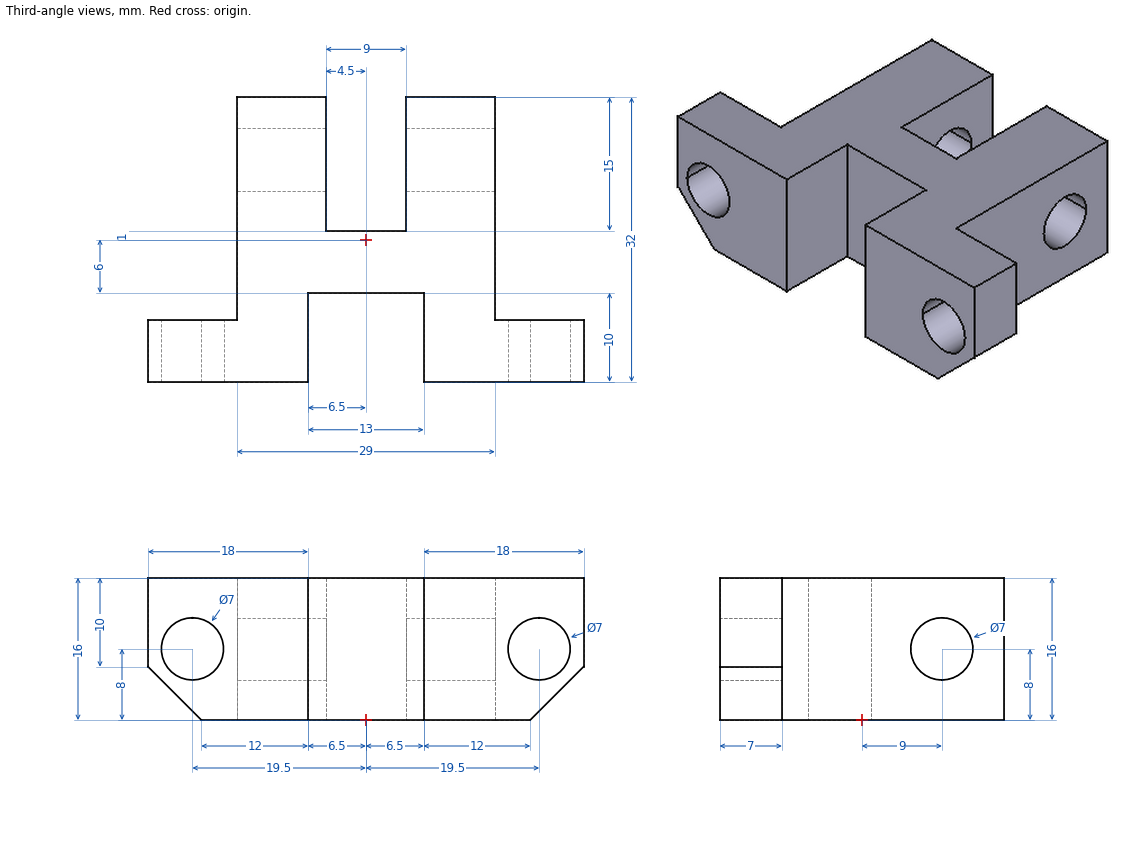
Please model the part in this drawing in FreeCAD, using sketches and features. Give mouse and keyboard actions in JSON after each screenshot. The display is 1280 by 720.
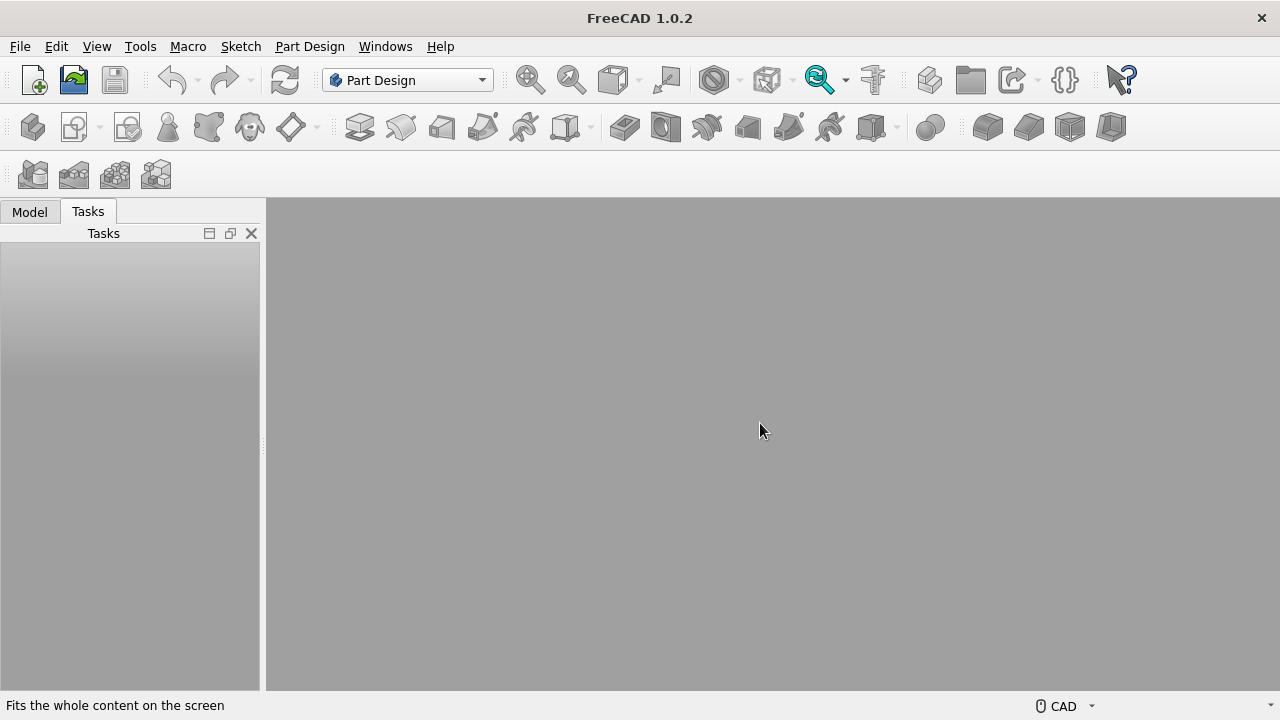
{"action": "left_click", "coordinate": [33, 80]}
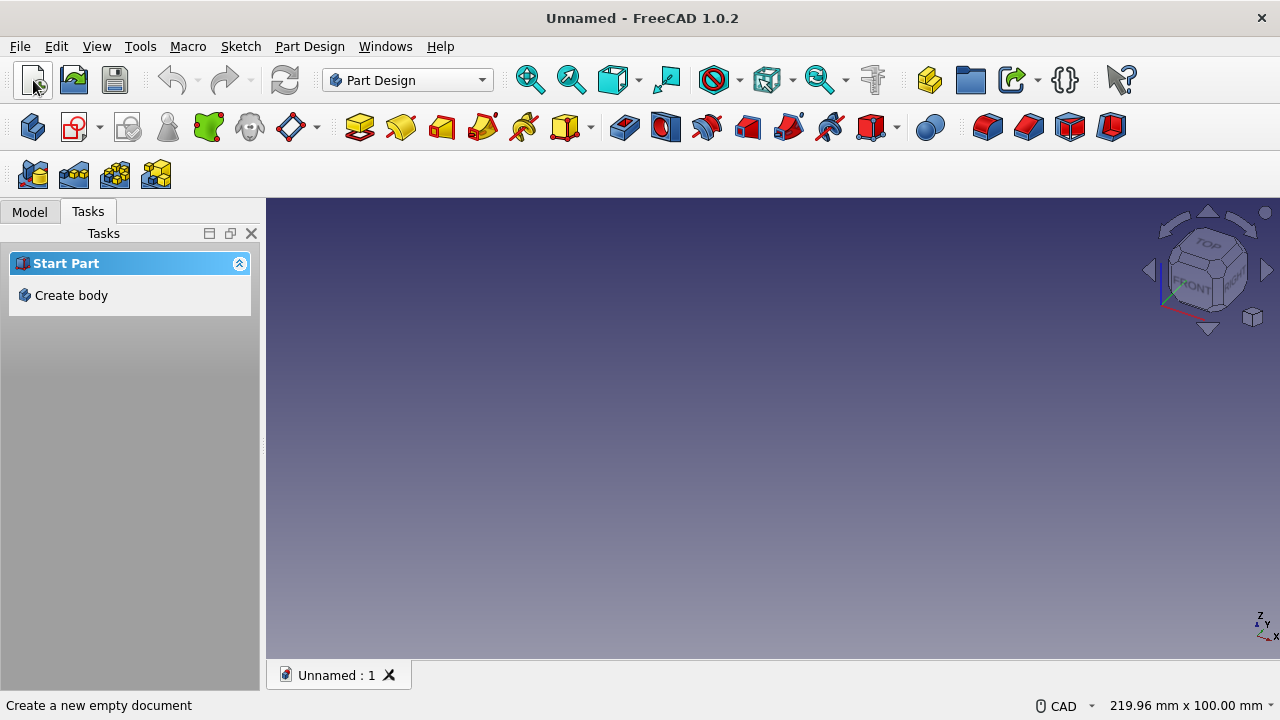
{"action": "left_click", "coordinate": [74, 128]}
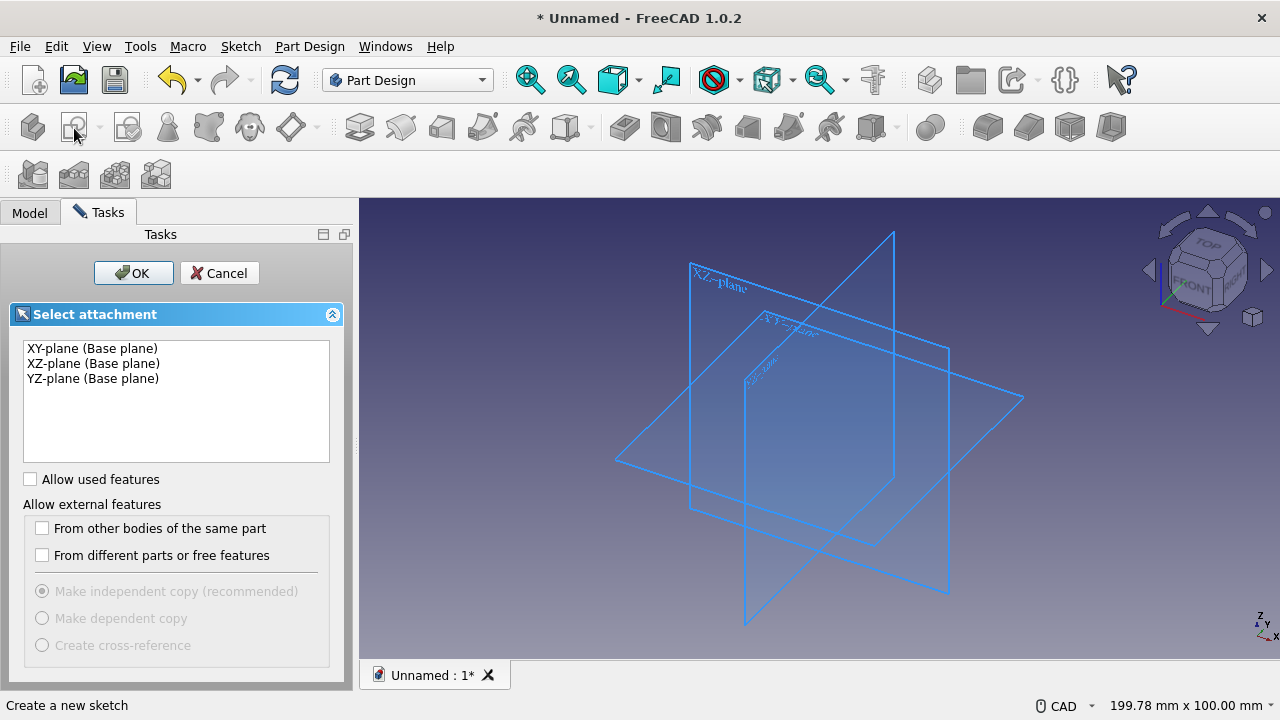
{"action": "left_click", "coordinate": [84, 348]}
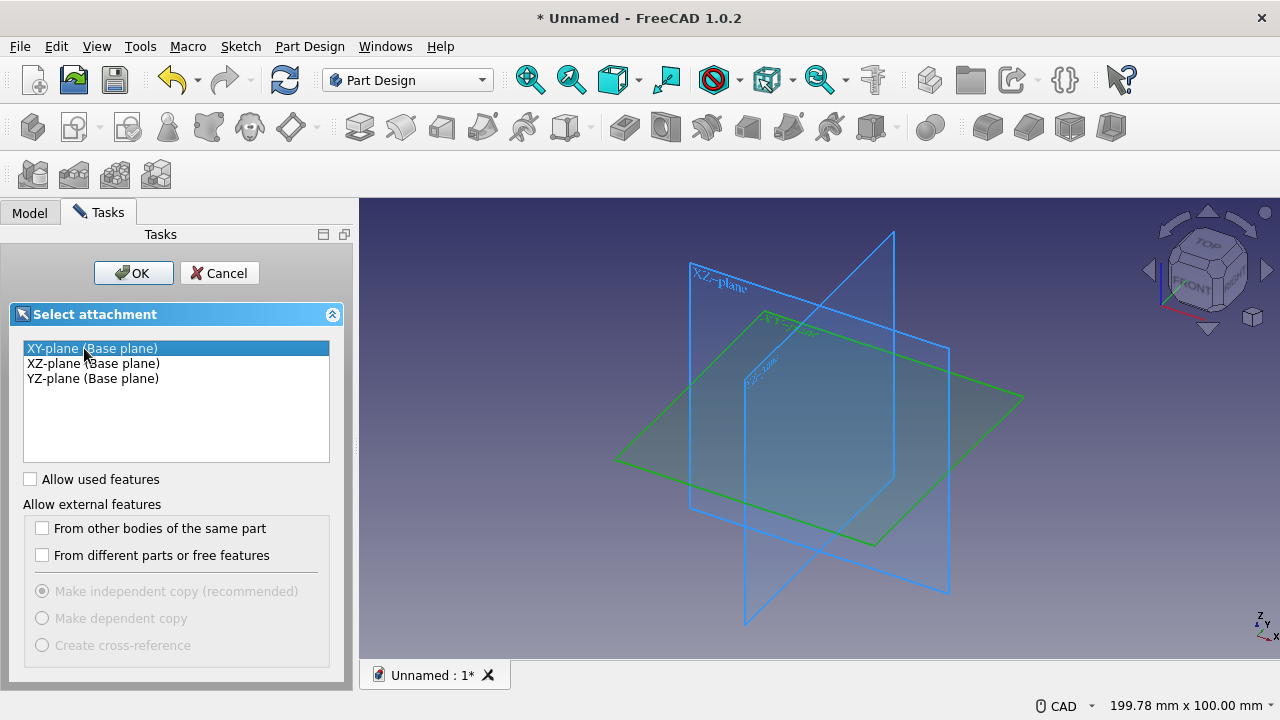
{"action": "left_click", "coordinate": [134, 273]}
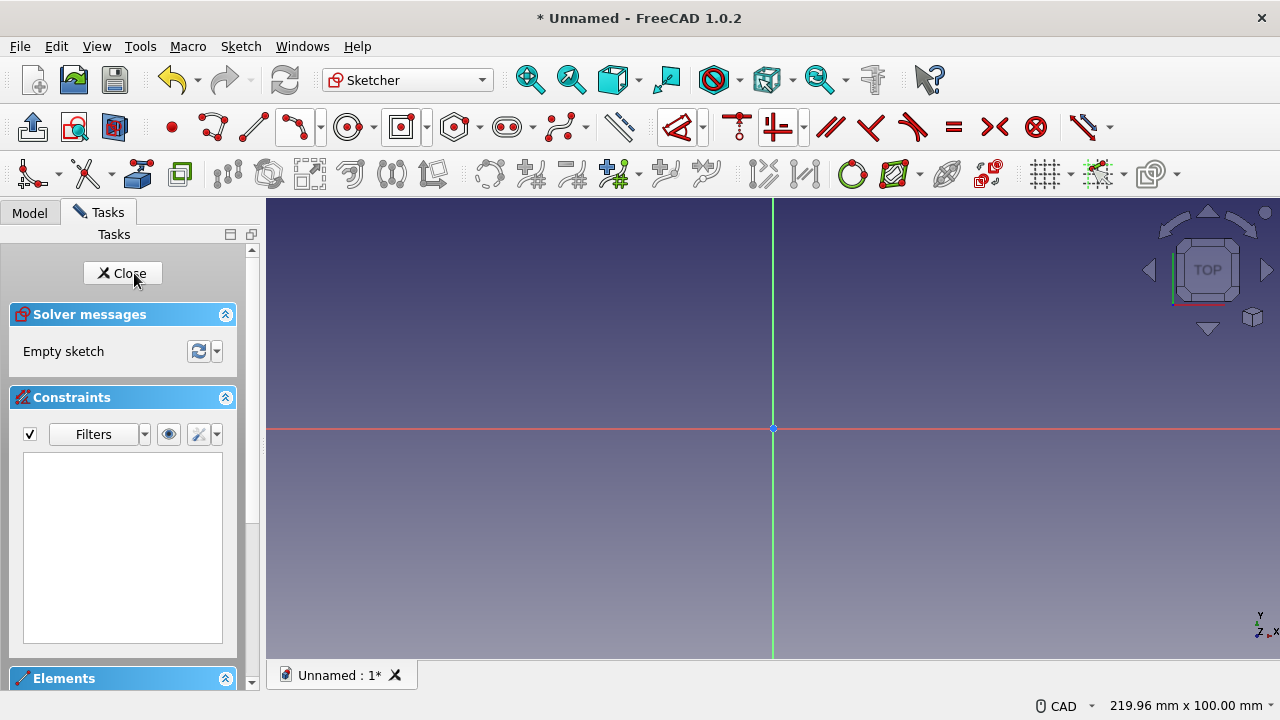
{"action": "scroll", "coordinate": [856, 428], "scroll_direction": "up", "scroll_amount": 3}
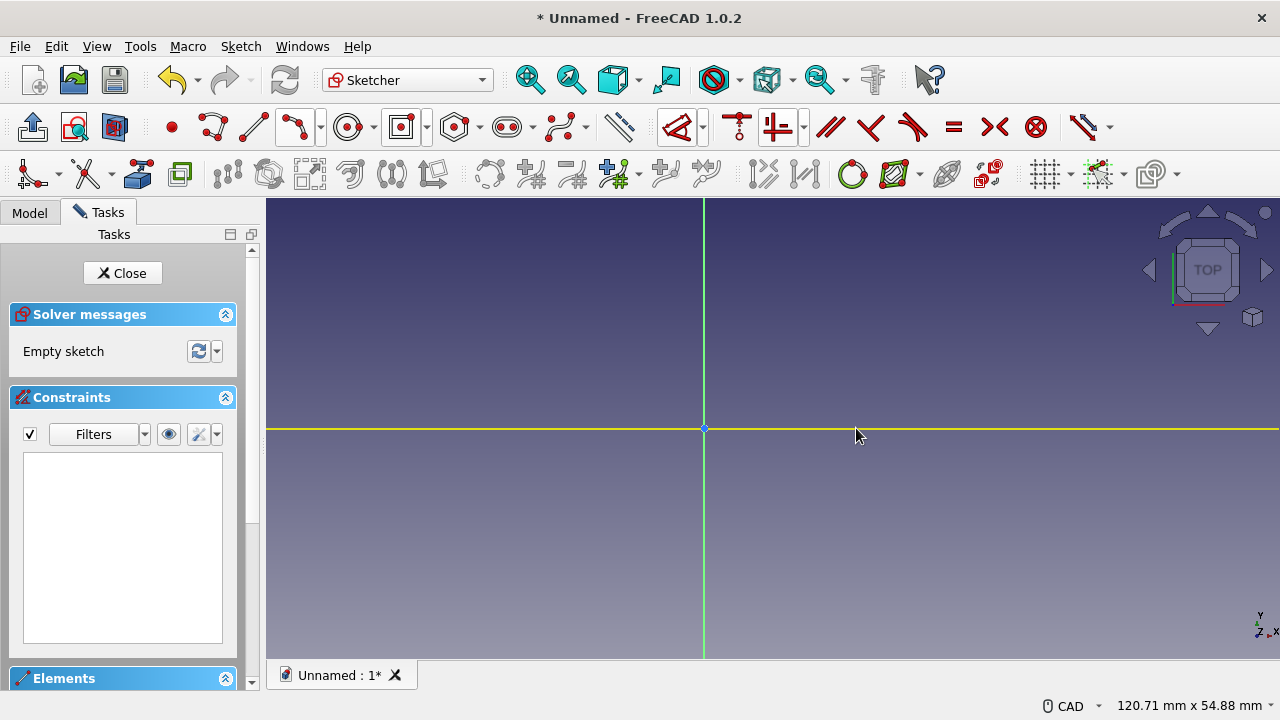
{"action": "left_click", "coordinate": [400, 128]}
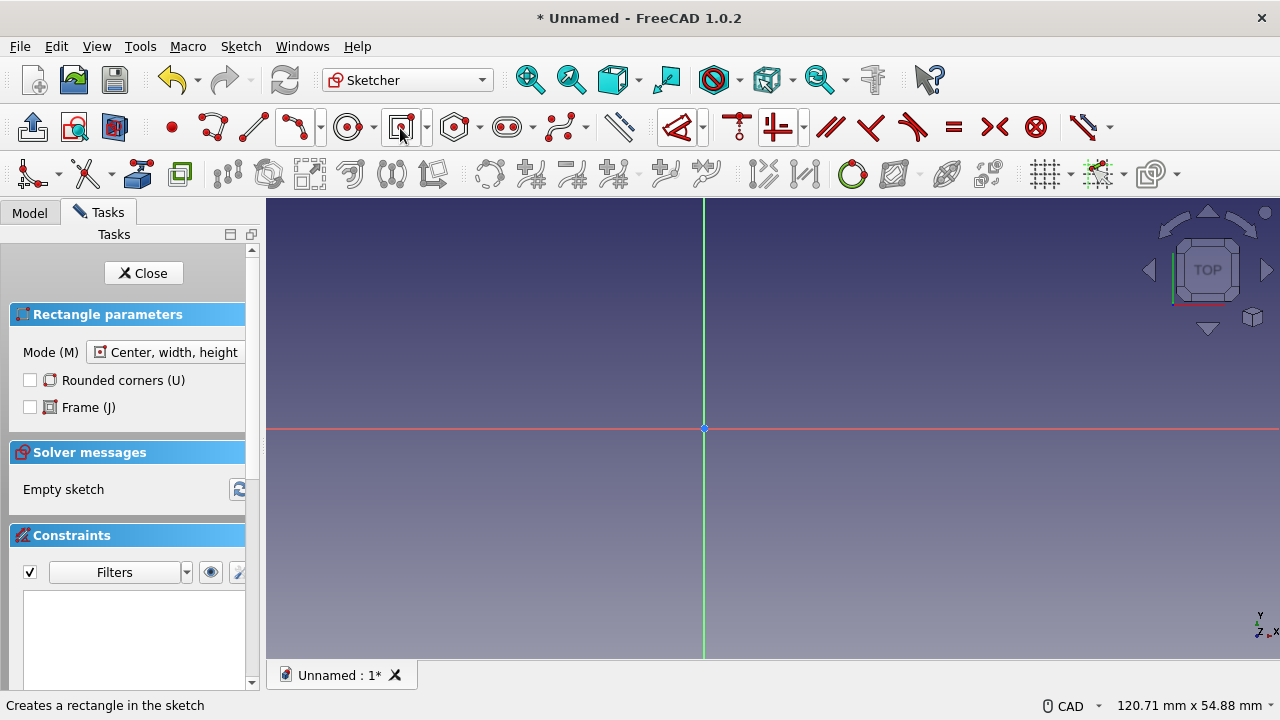
{"action": "left_click", "coordinate": [704, 428]}
{"action": "mouse_move", "coordinate": [826, 294]}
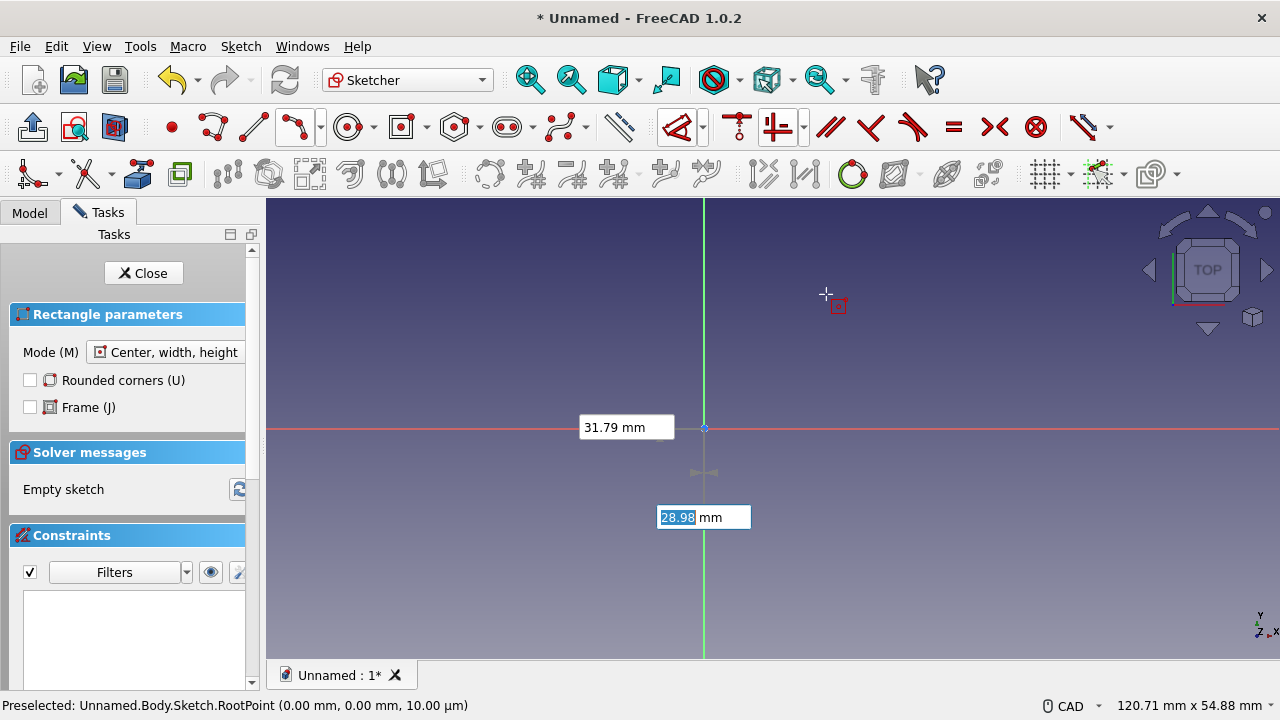
{"action": "type", "text": "29"}
{"action": "key", "text": "Tab"}
{"action": "type", "text": "32"}
{"action": "key", "text": "Return"}
{"action": "key", "text": "Escape"}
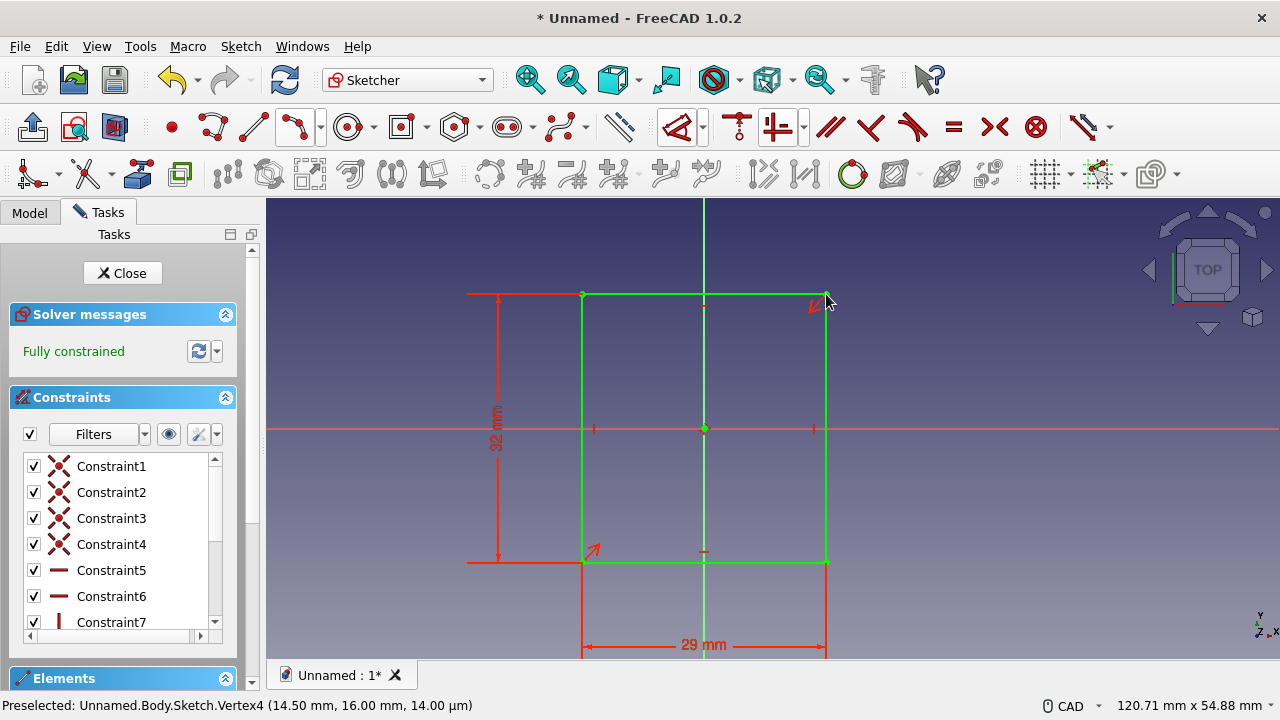
{"action": "left_click", "coordinate": [123, 273]}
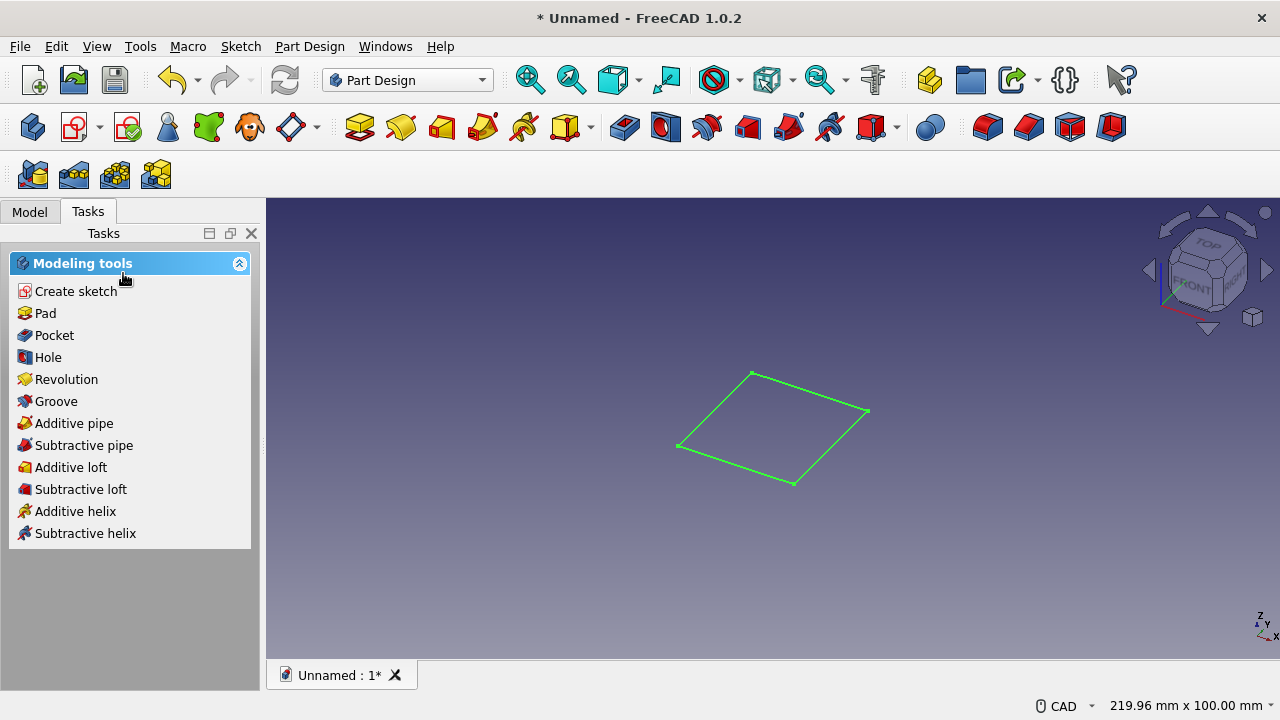
{"action": "left_click", "coordinate": [360, 128]}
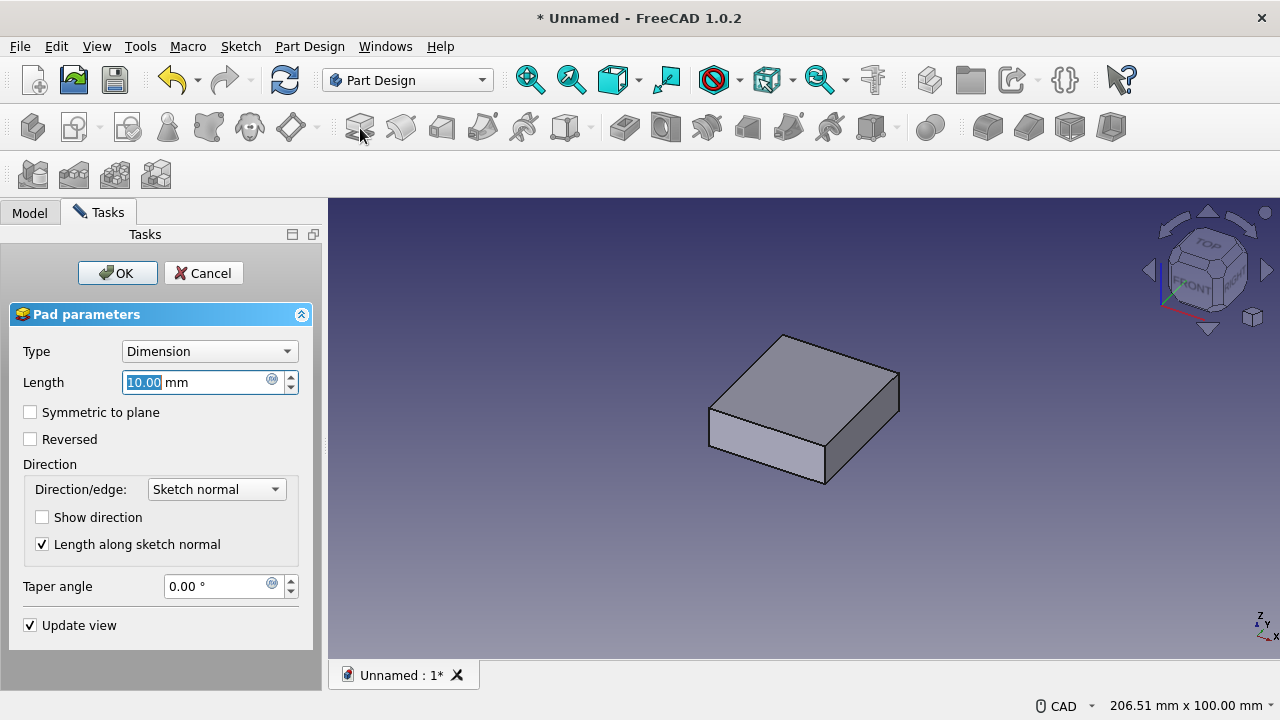
{"action": "type", "text": "16"}
{"action": "key", "text": "Tab"}